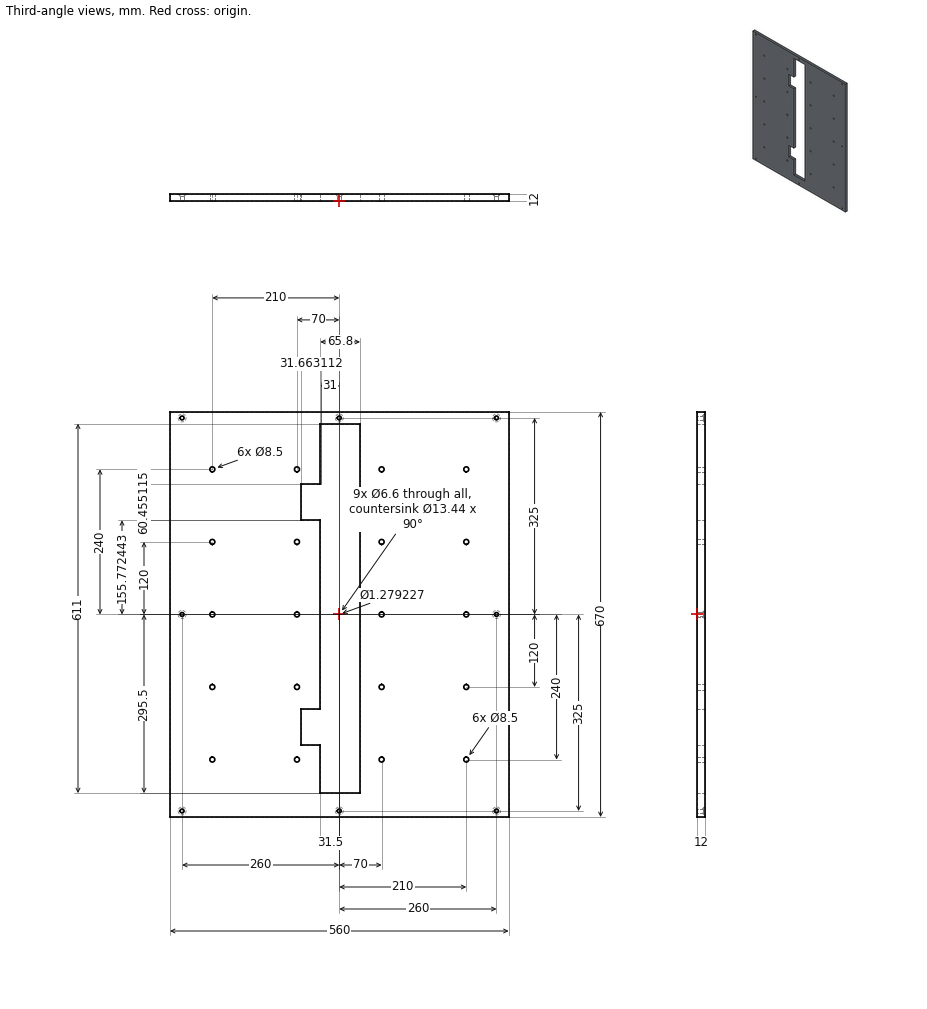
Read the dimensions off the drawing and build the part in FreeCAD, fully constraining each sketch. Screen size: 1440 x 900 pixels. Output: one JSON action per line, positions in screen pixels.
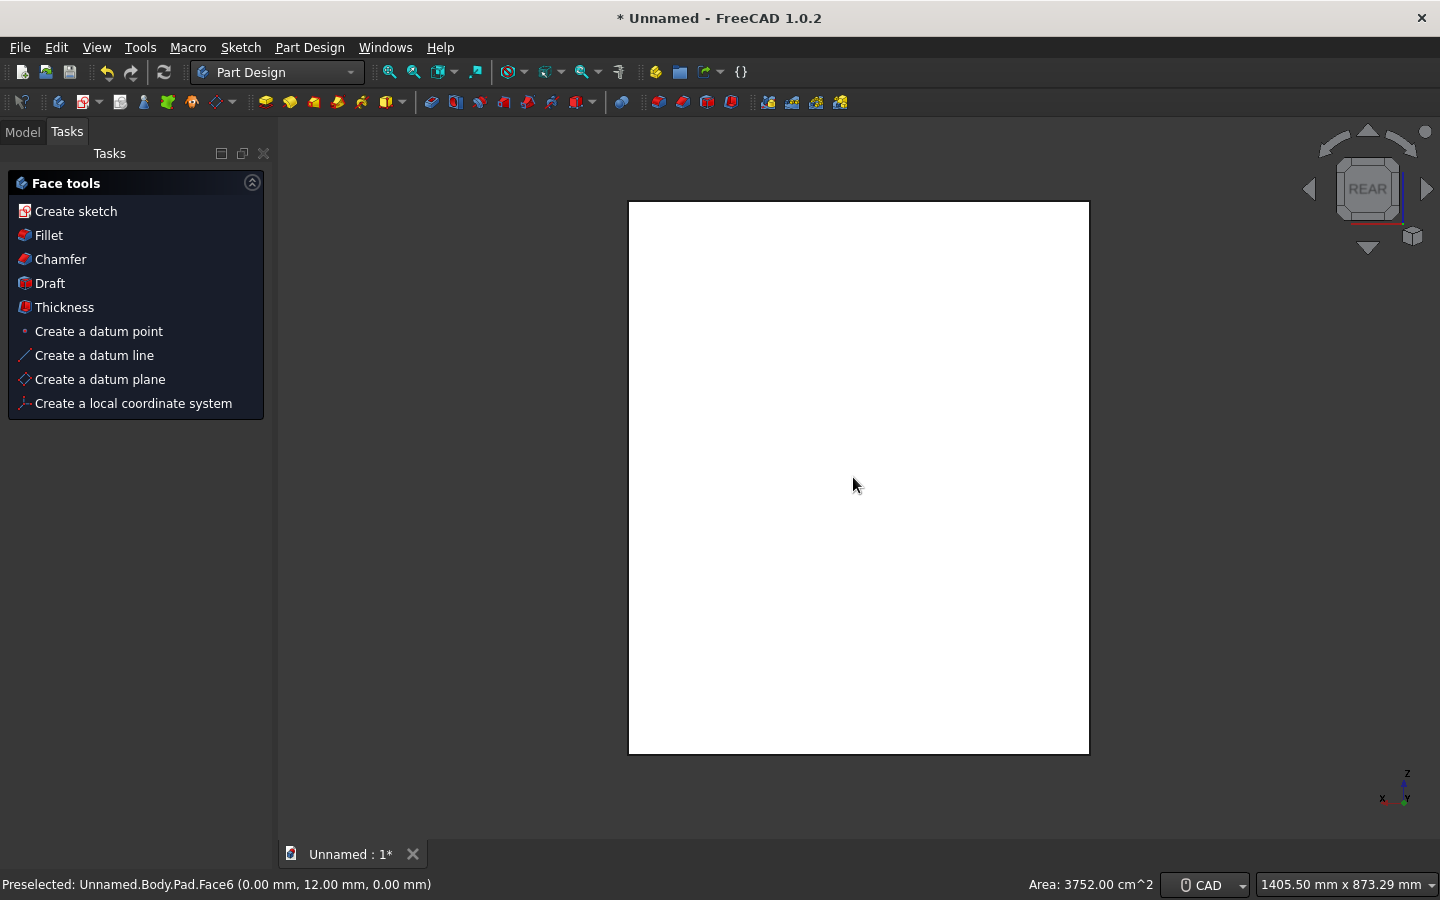
{"action": "left_click", "coordinate": [84, 102]}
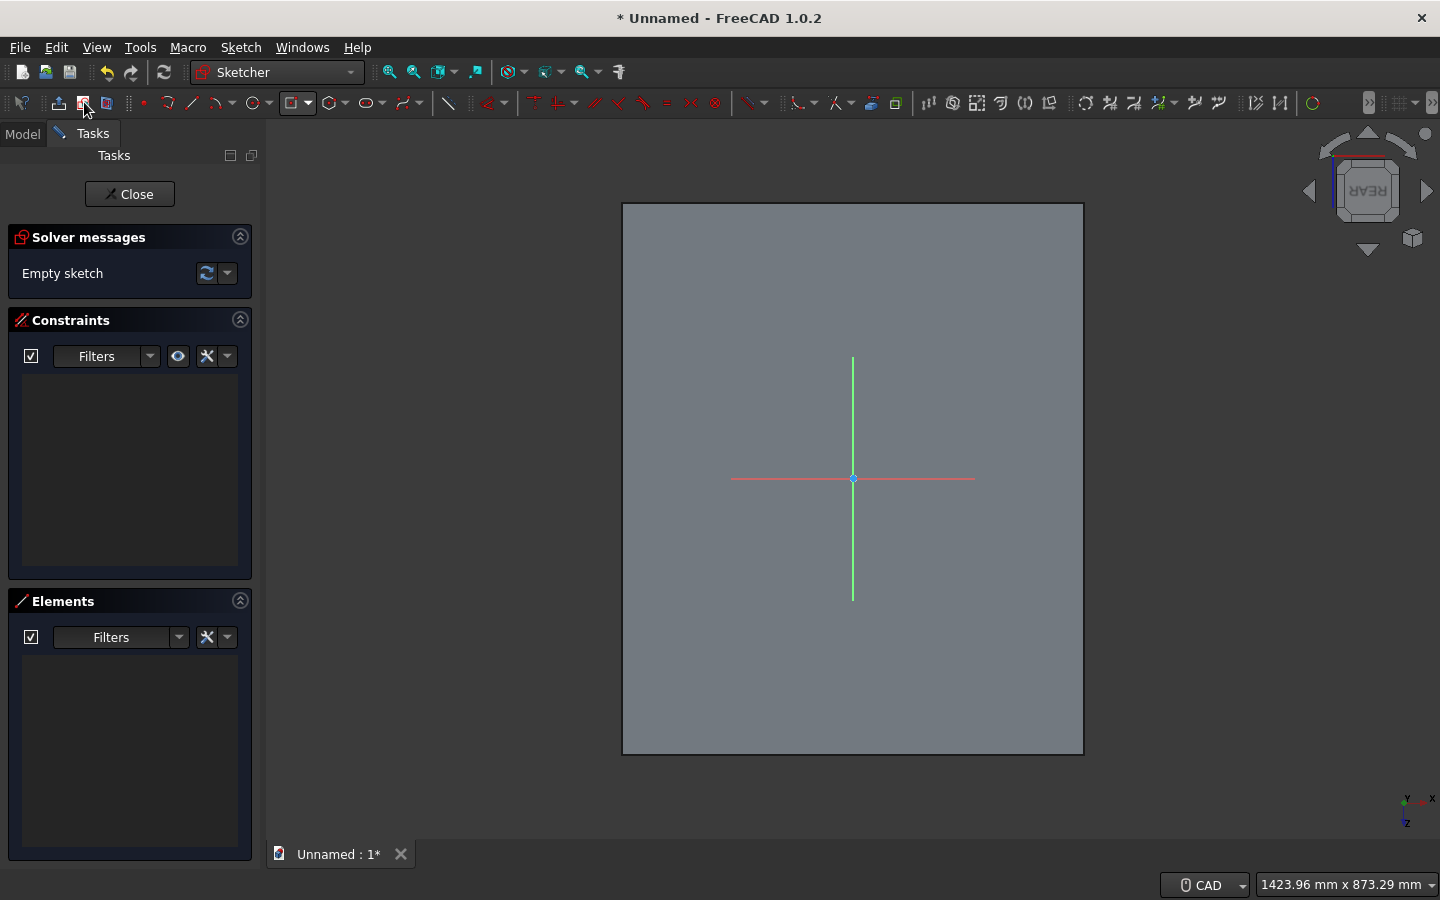
{"action": "scroll", "coordinate": [1069, 299], "scroll_direction": "up", "scroll_amount": 4}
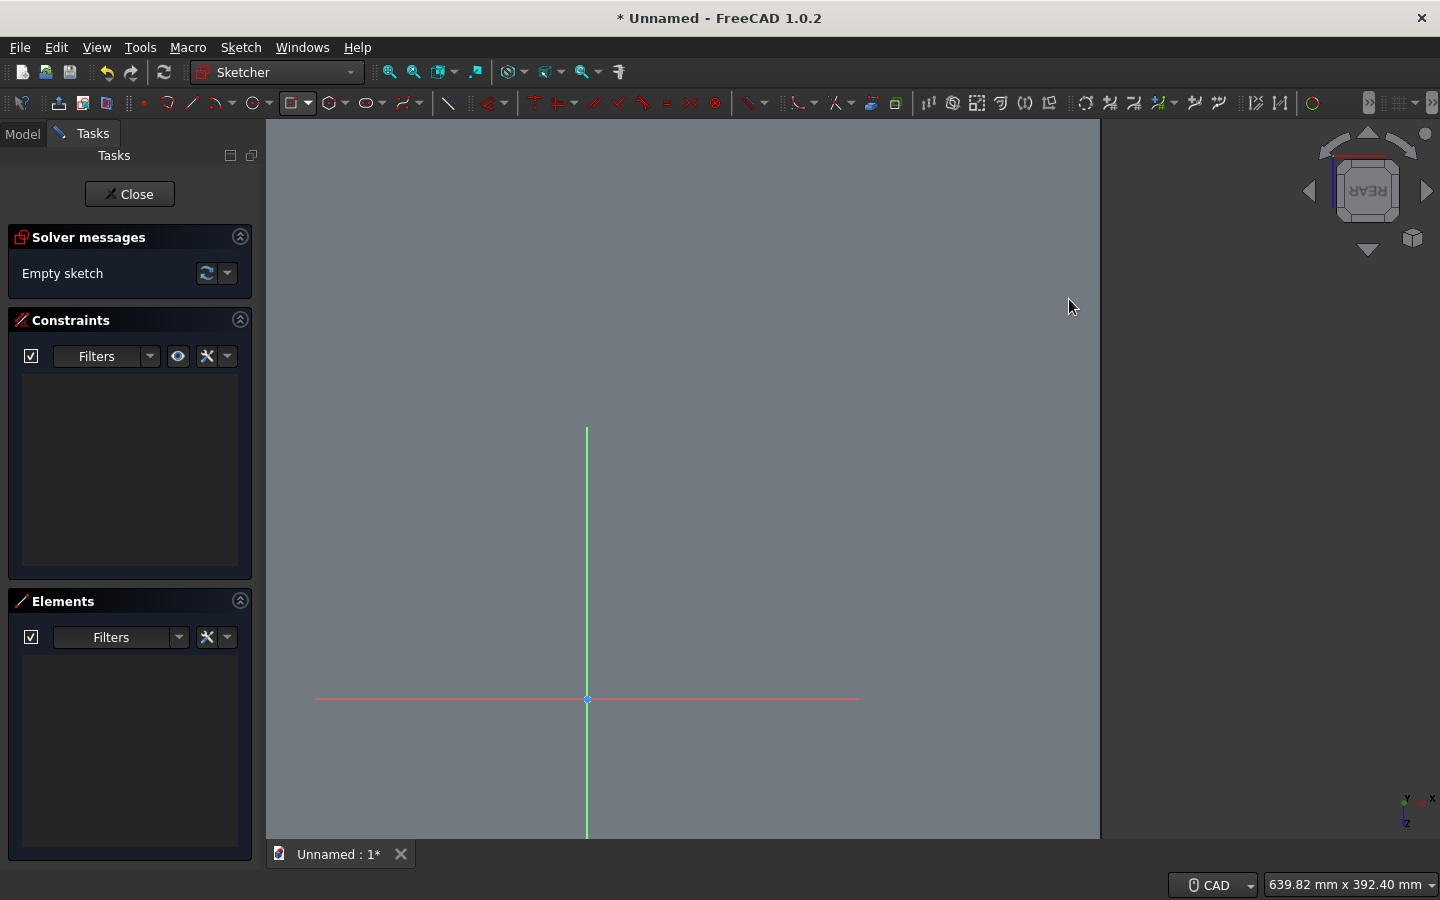
{"action": "left_click", "coordinate": [254, 104]}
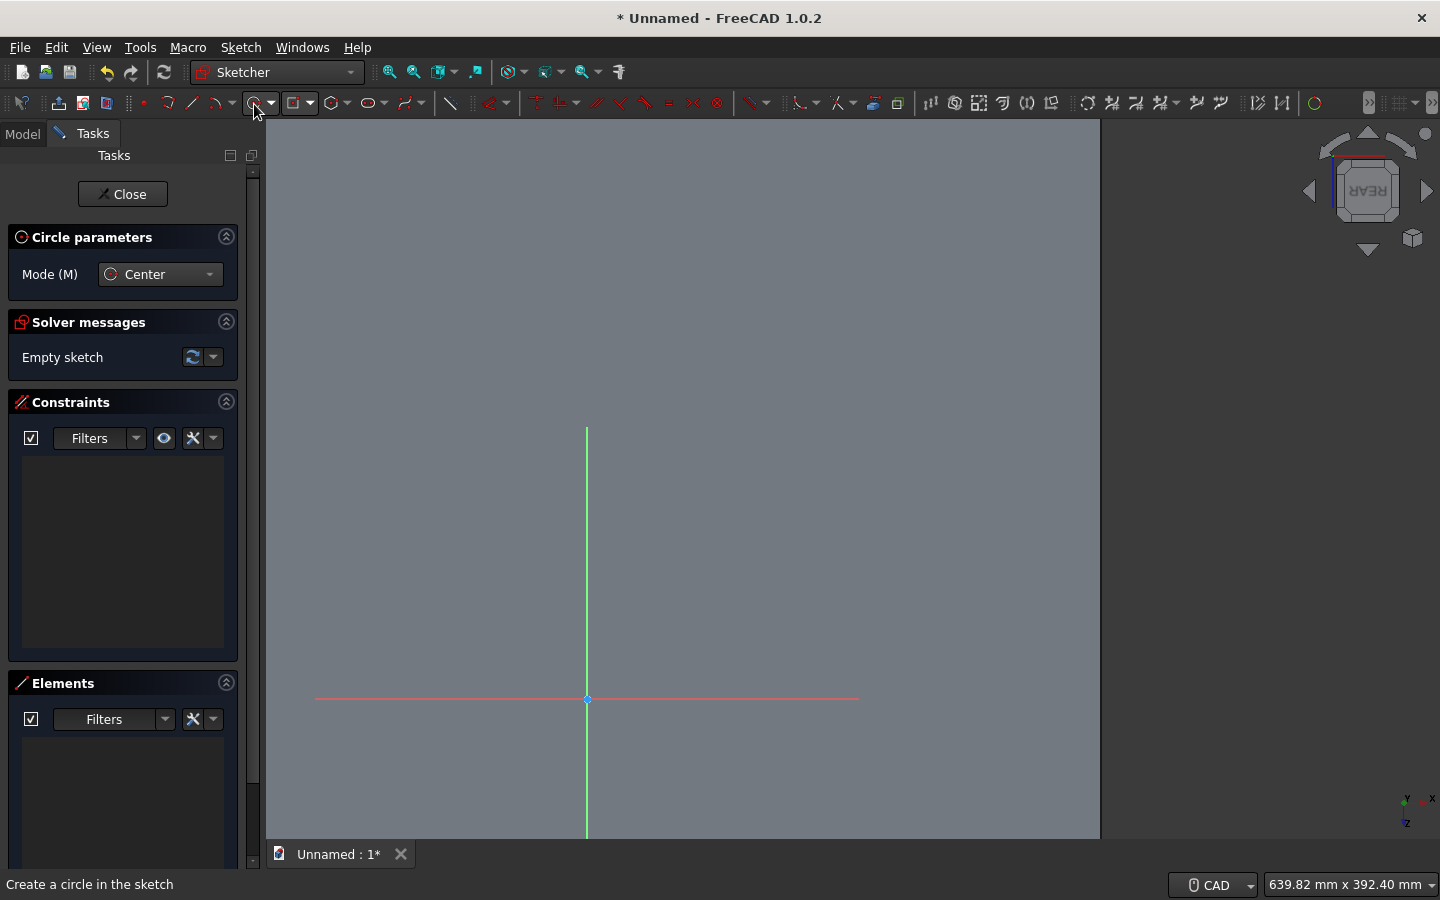
{"action": "scroll", "coordinate": [973, 259], "scroll_direction": "up", "scroll_amount": 6}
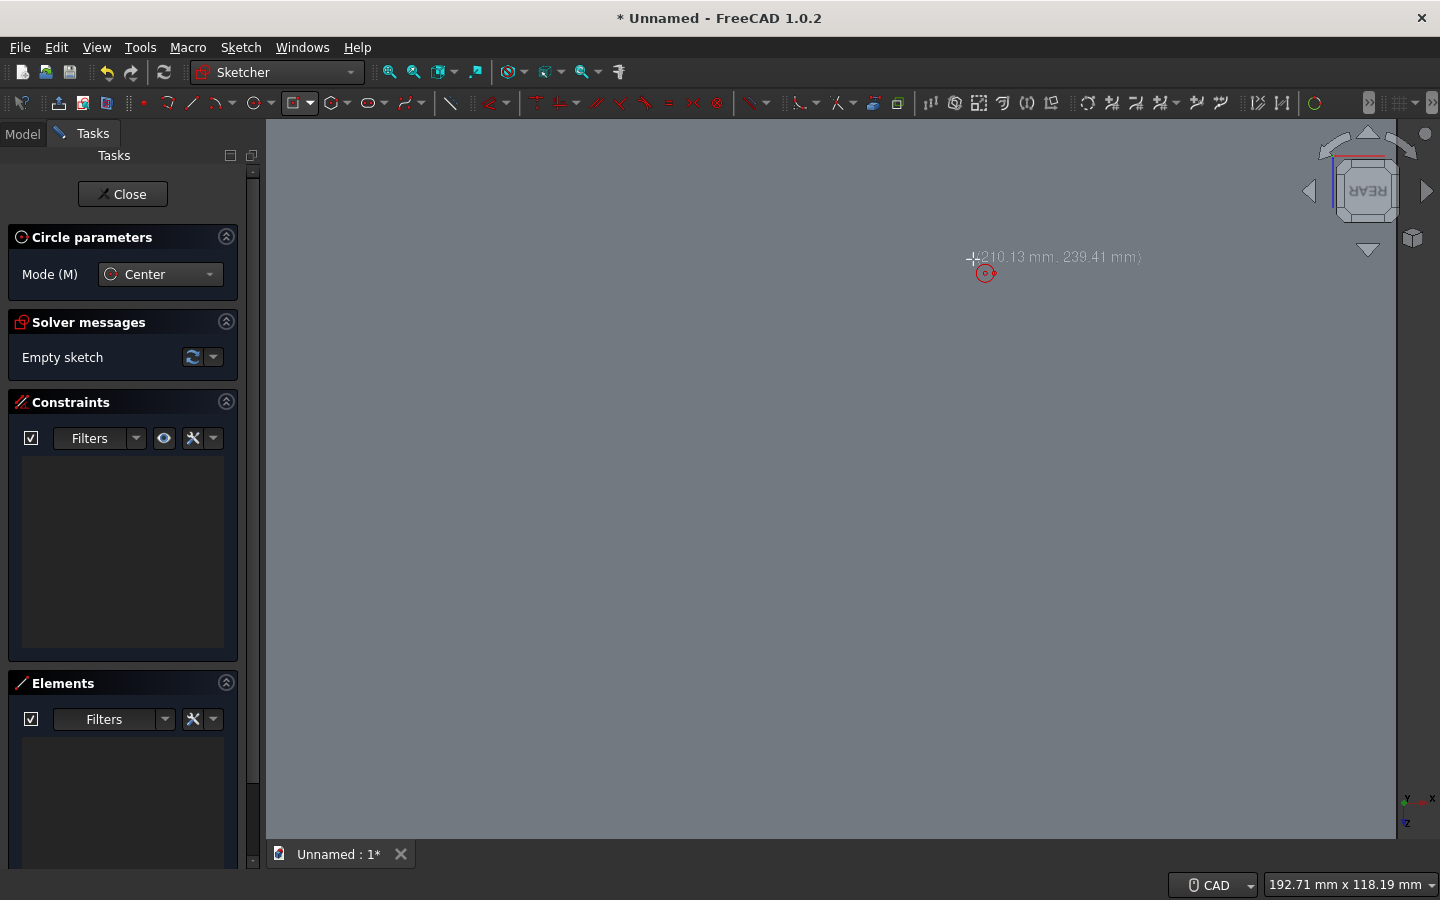
{"action": "left_click", "coordinate": [971, 258]}
{"action": "left_click", "coordinate": [989, 240]}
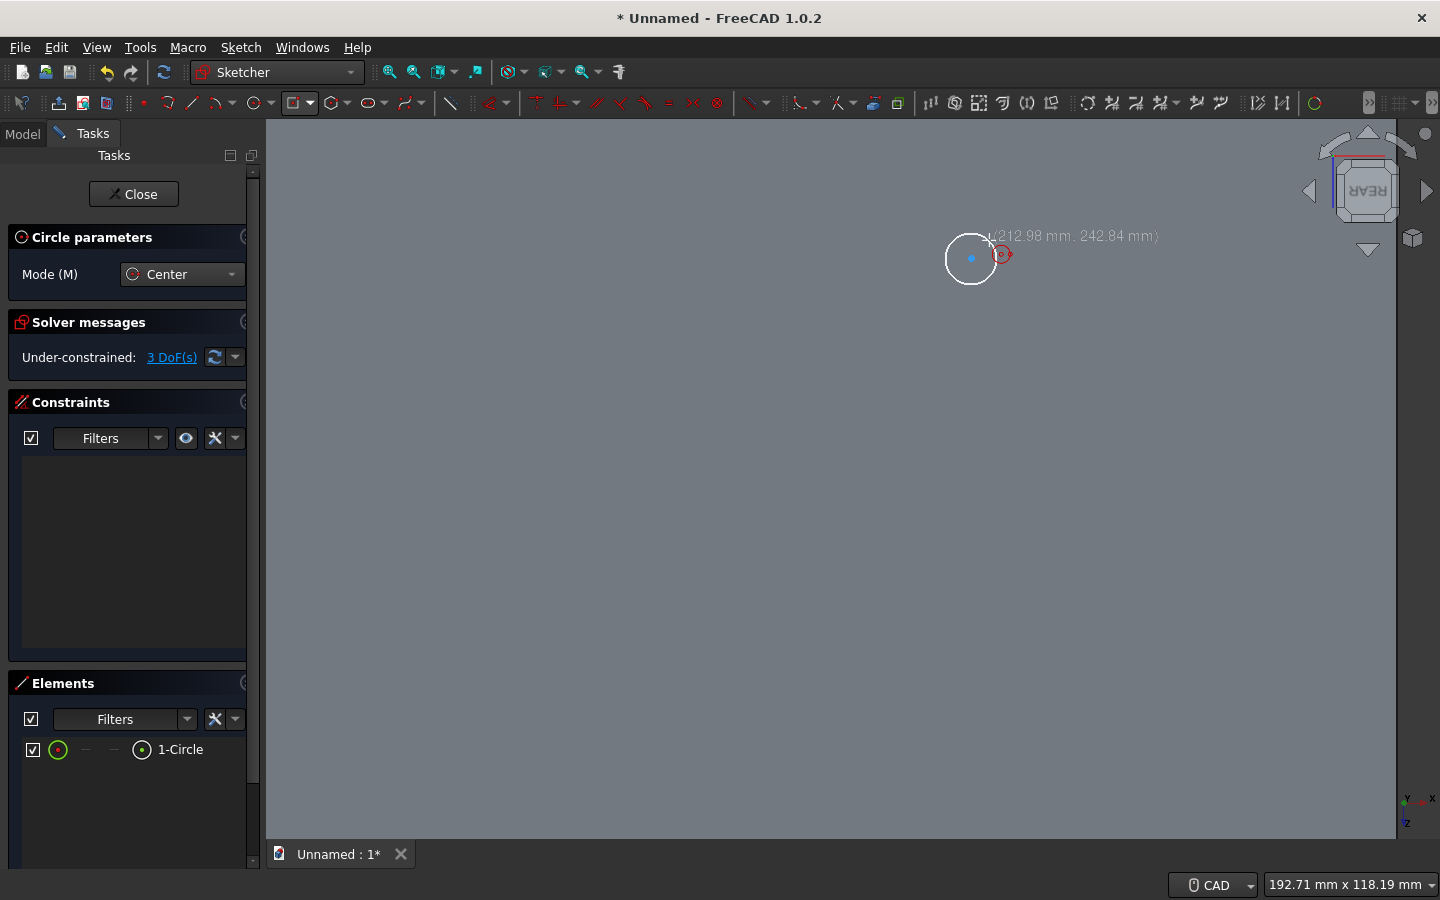
{"action": "scroll", "coordinate": [975, 259], "scroll_direction": "down", "scroll_amount": 6}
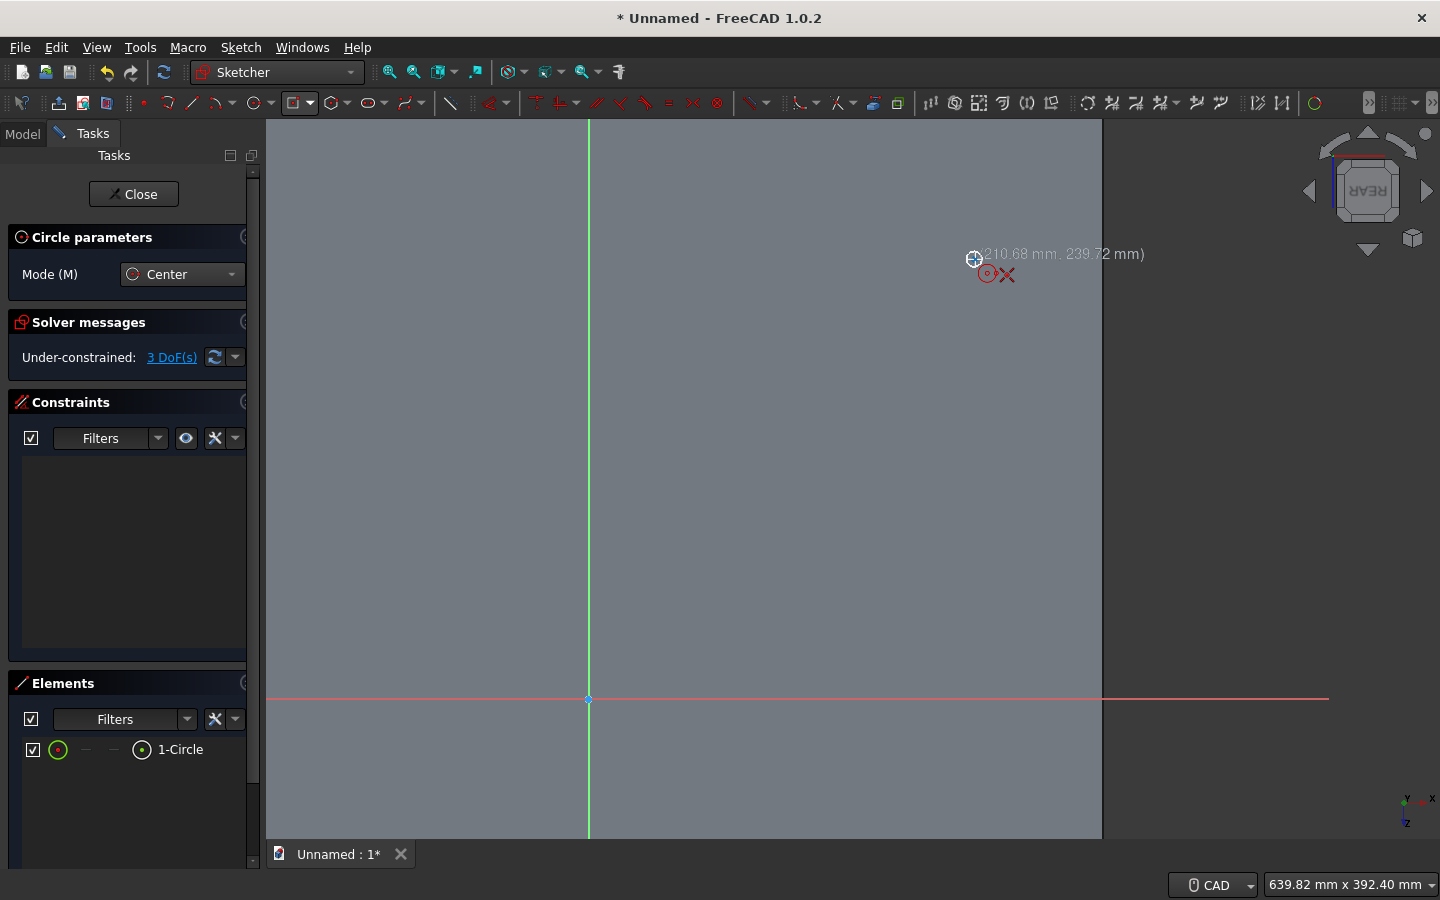
{"action": "scroll", "coordinate": [717, 259], "scroll_direction": "up", "scroll_amount": 6}